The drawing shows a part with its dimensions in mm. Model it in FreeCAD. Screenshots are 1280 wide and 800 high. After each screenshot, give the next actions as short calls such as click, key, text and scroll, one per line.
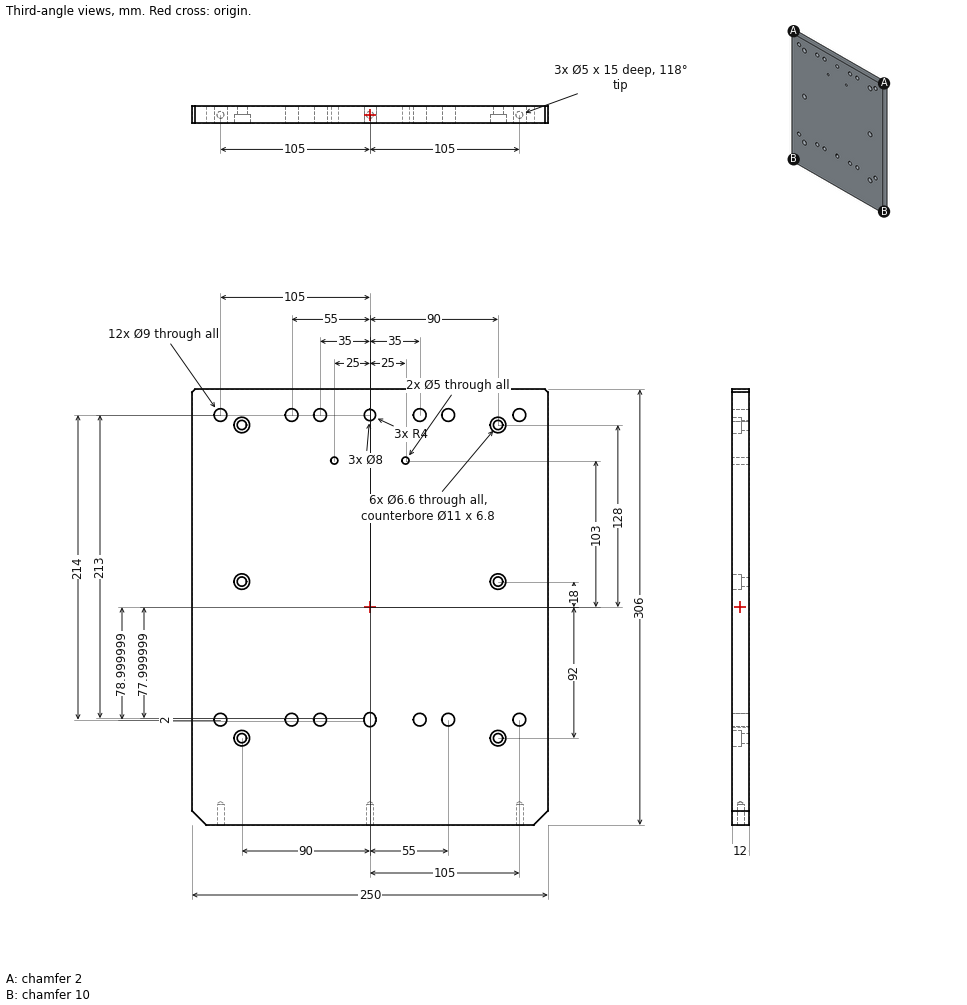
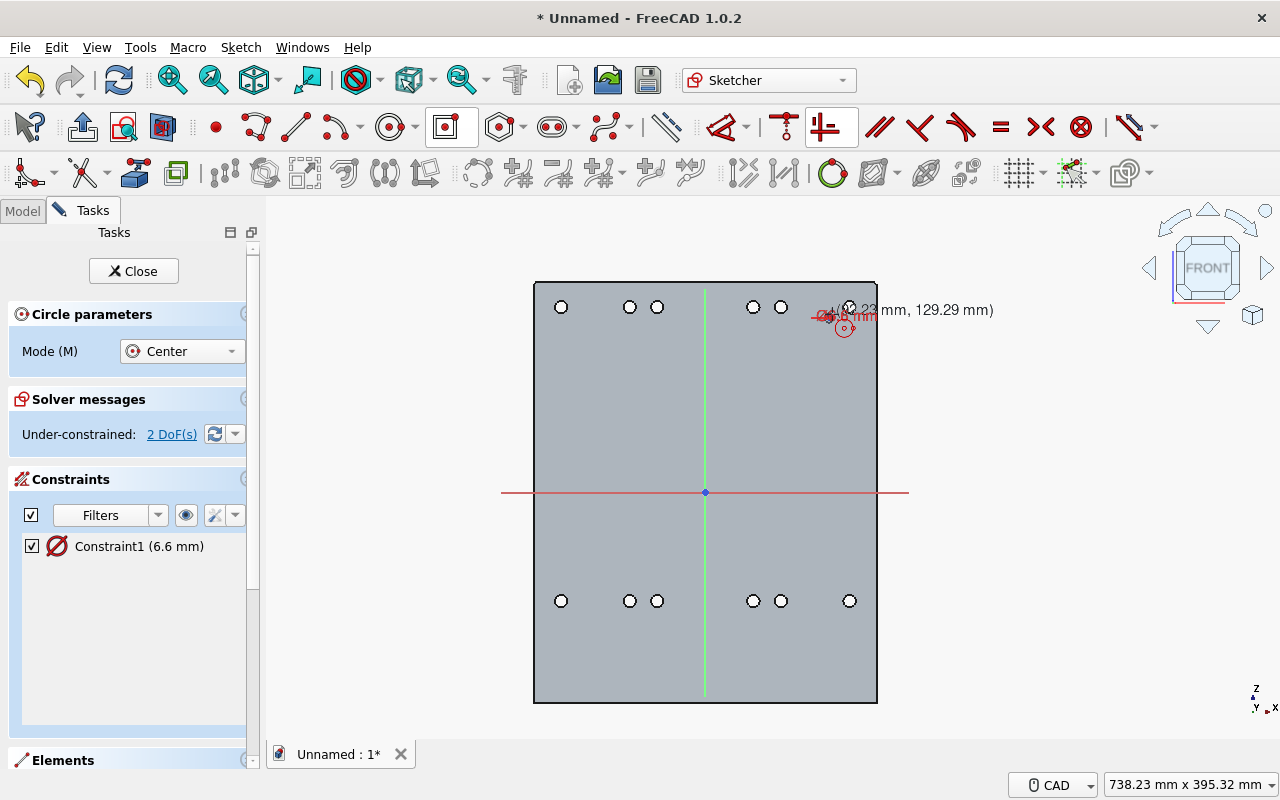
scroll(829, 468, up, 9)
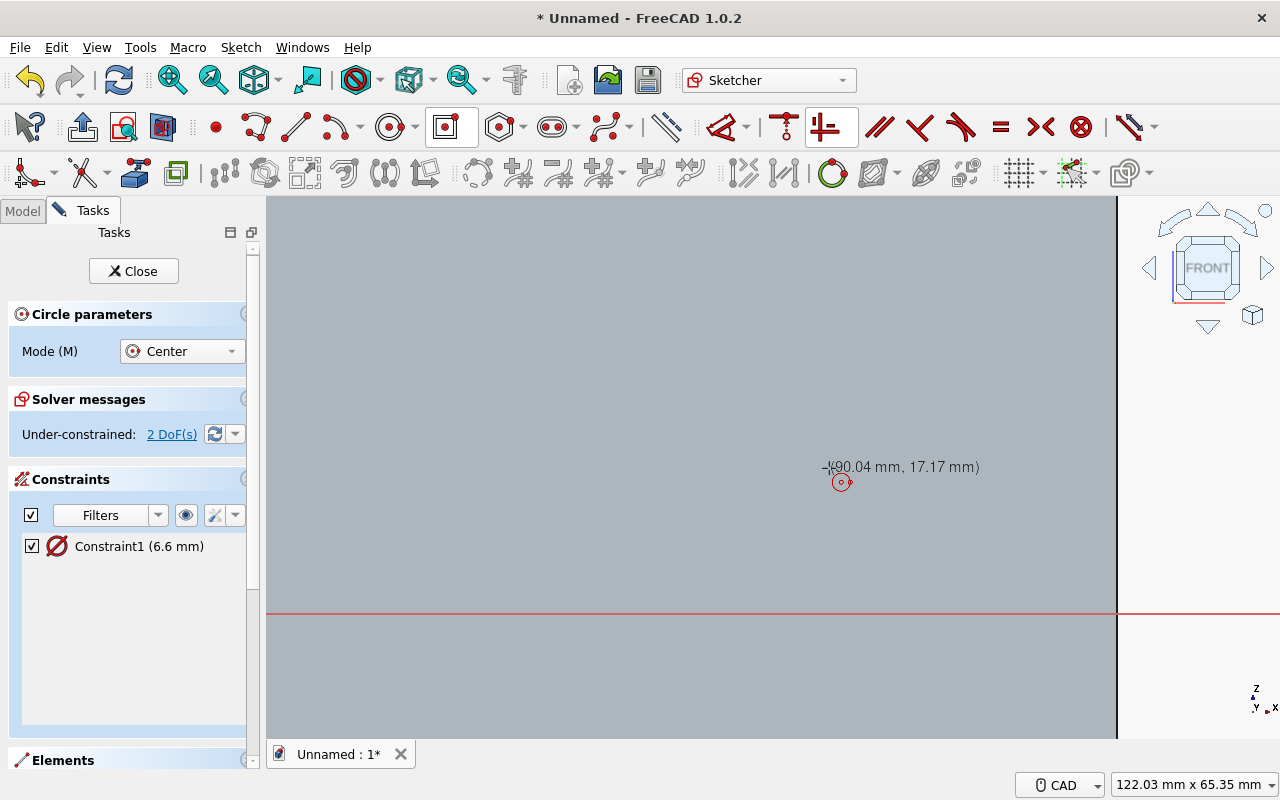
scroll(829, 468, down, 9)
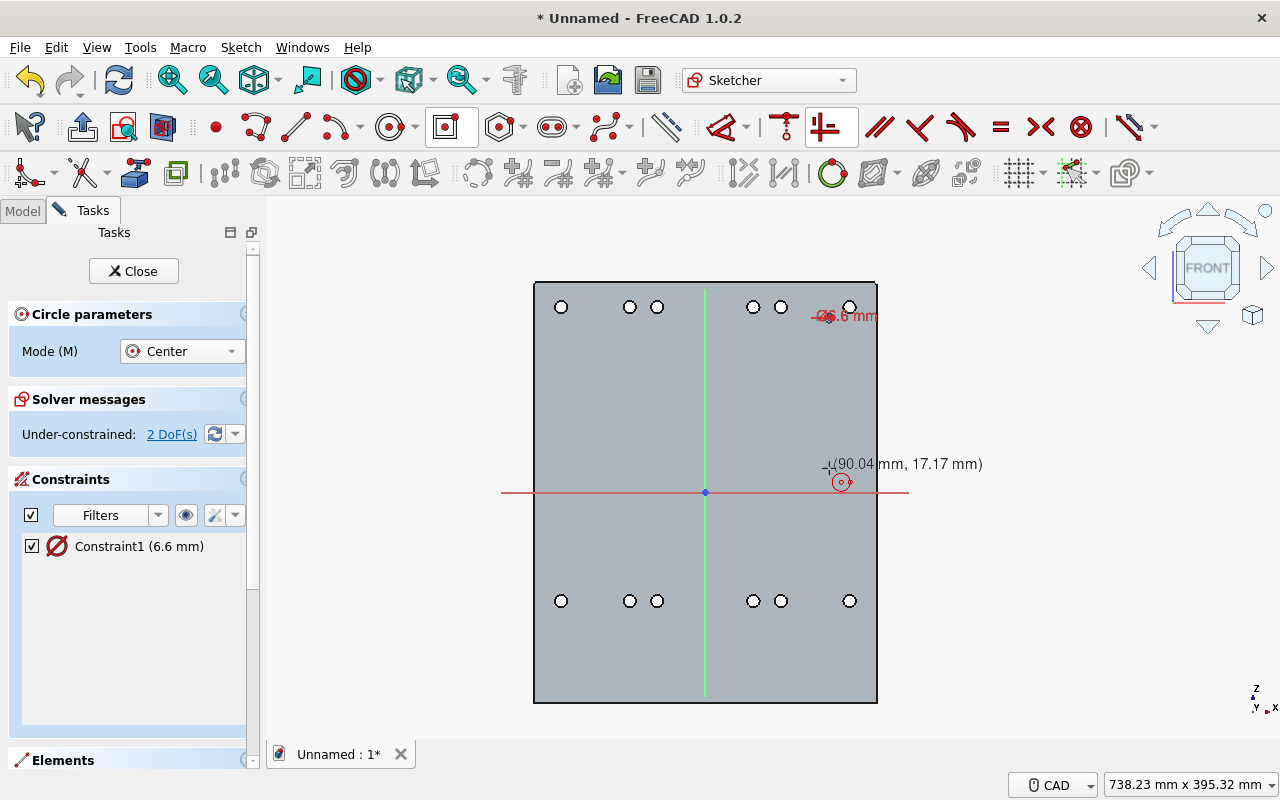
click(829, 468)
move(832, 465)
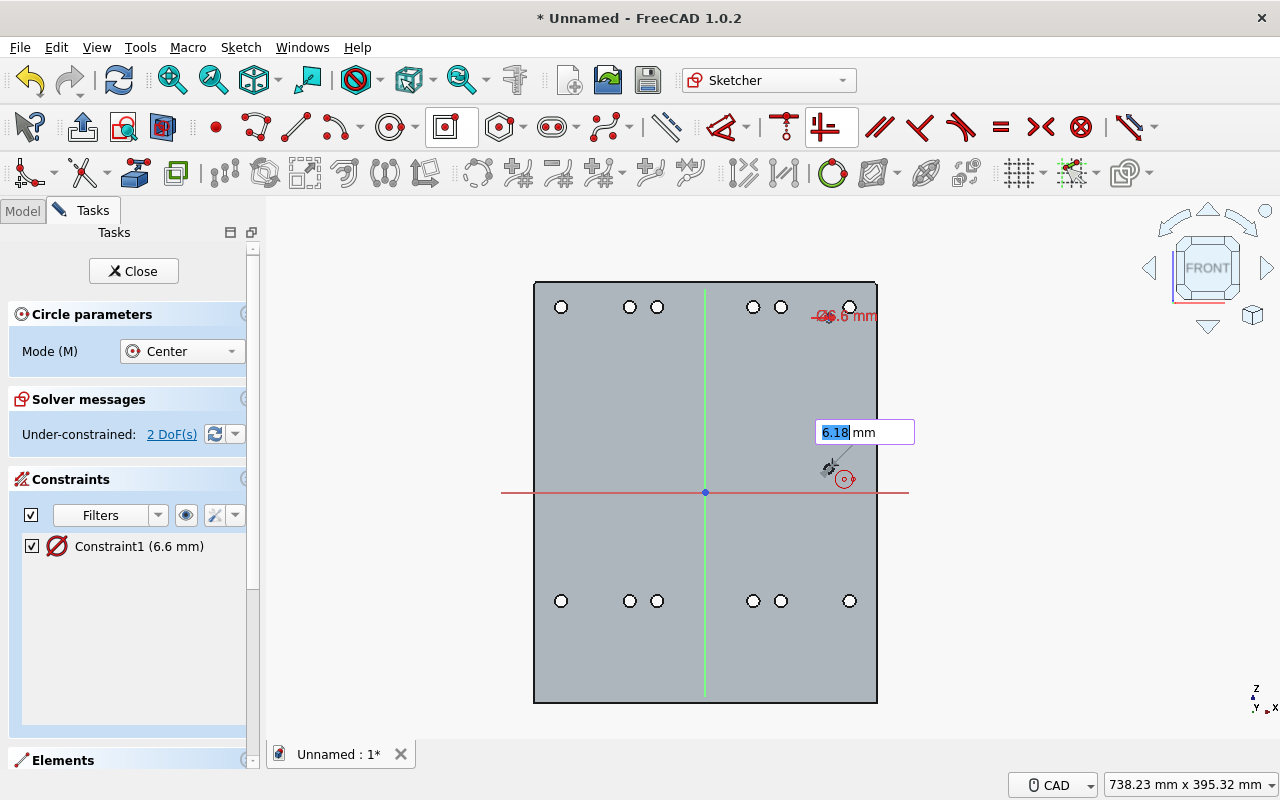
text(6.6)
key(Return)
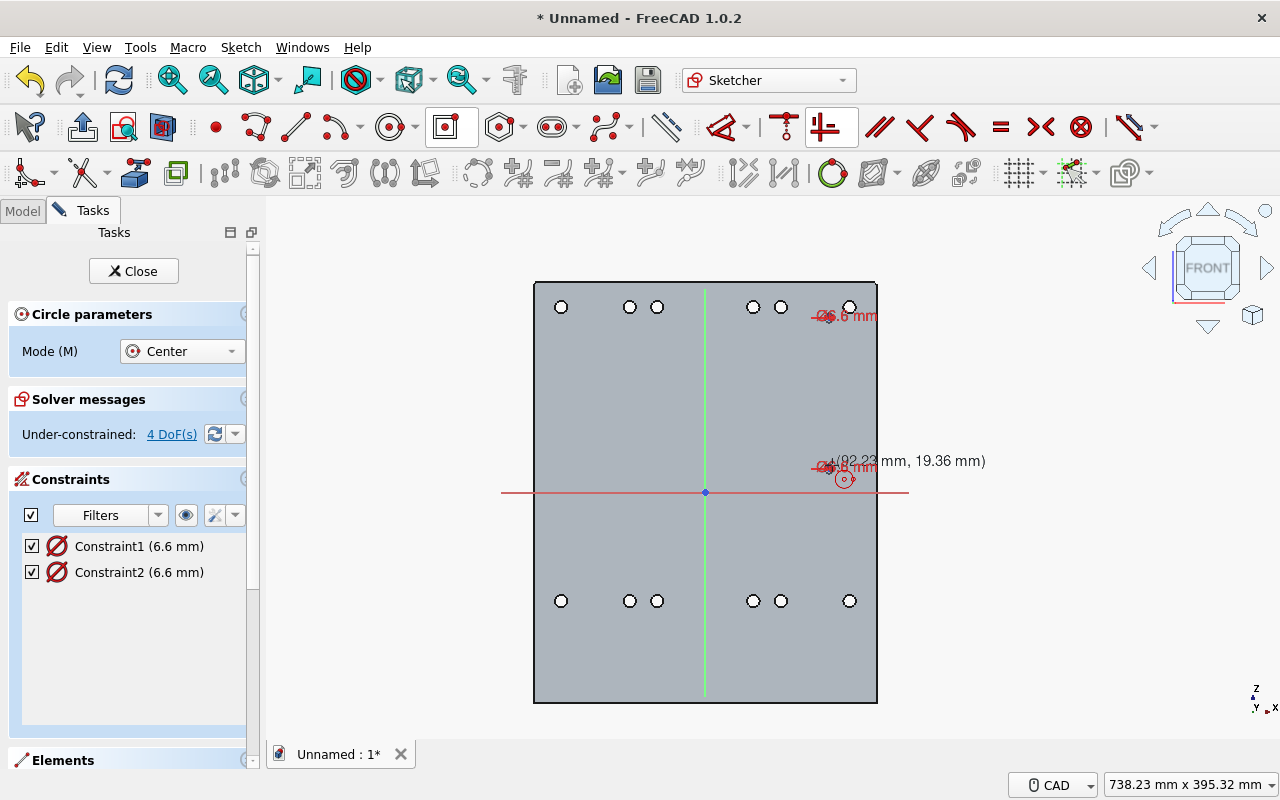
scroll(829, 619, up, 9)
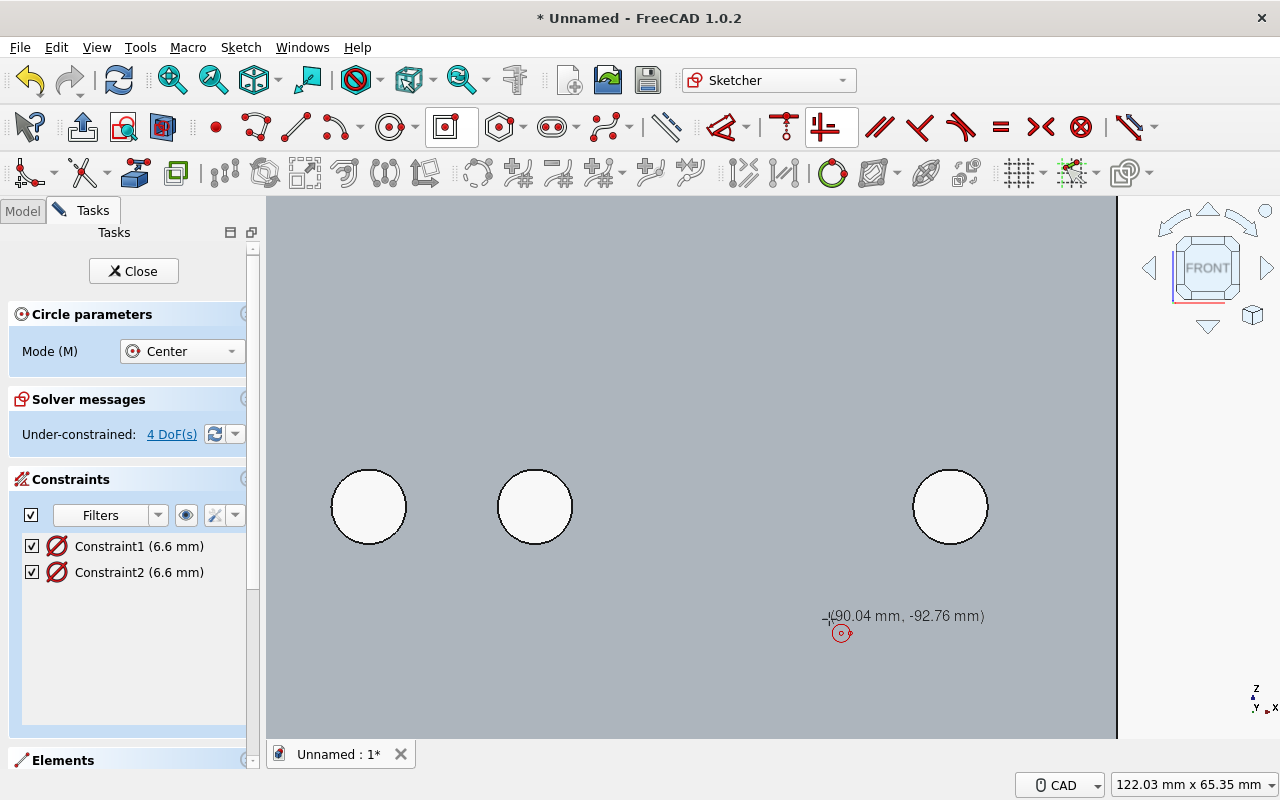
scroll(829, 619, down, 9)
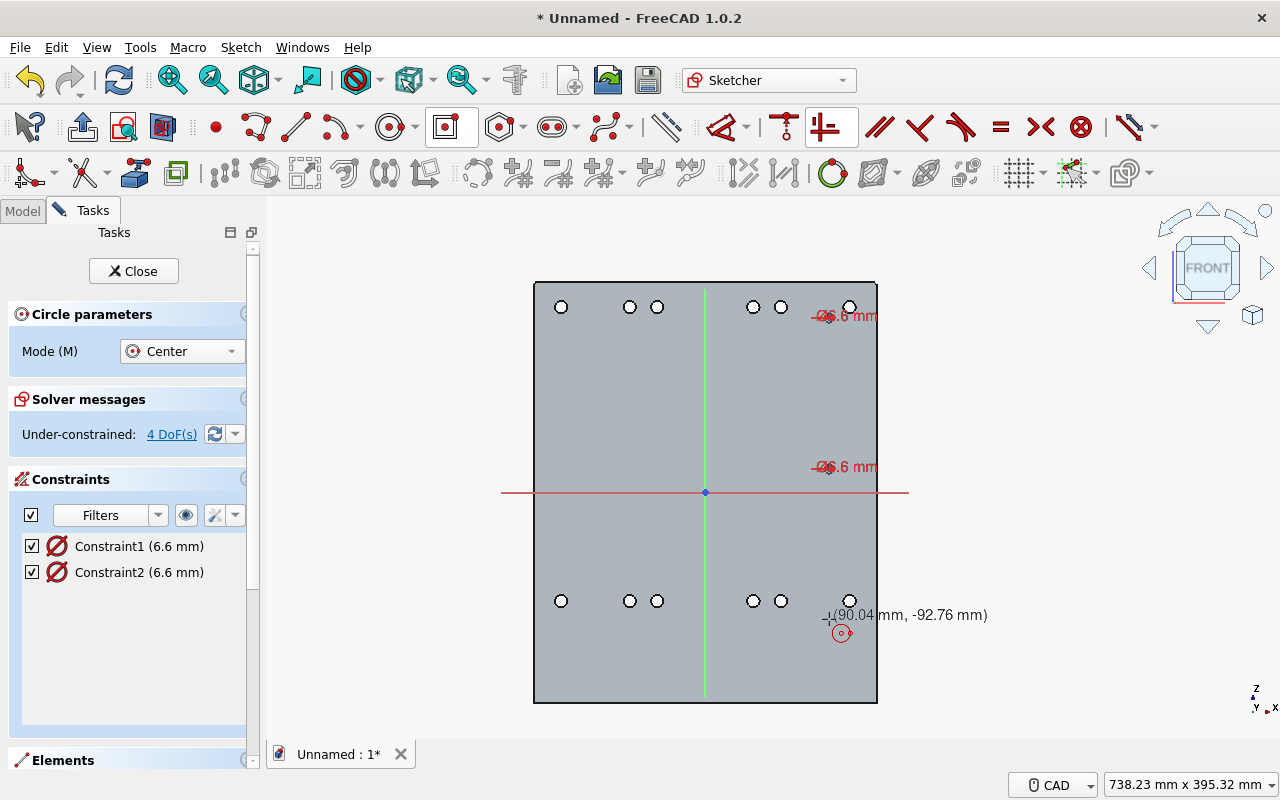
click(829, 619)
move(832, 616)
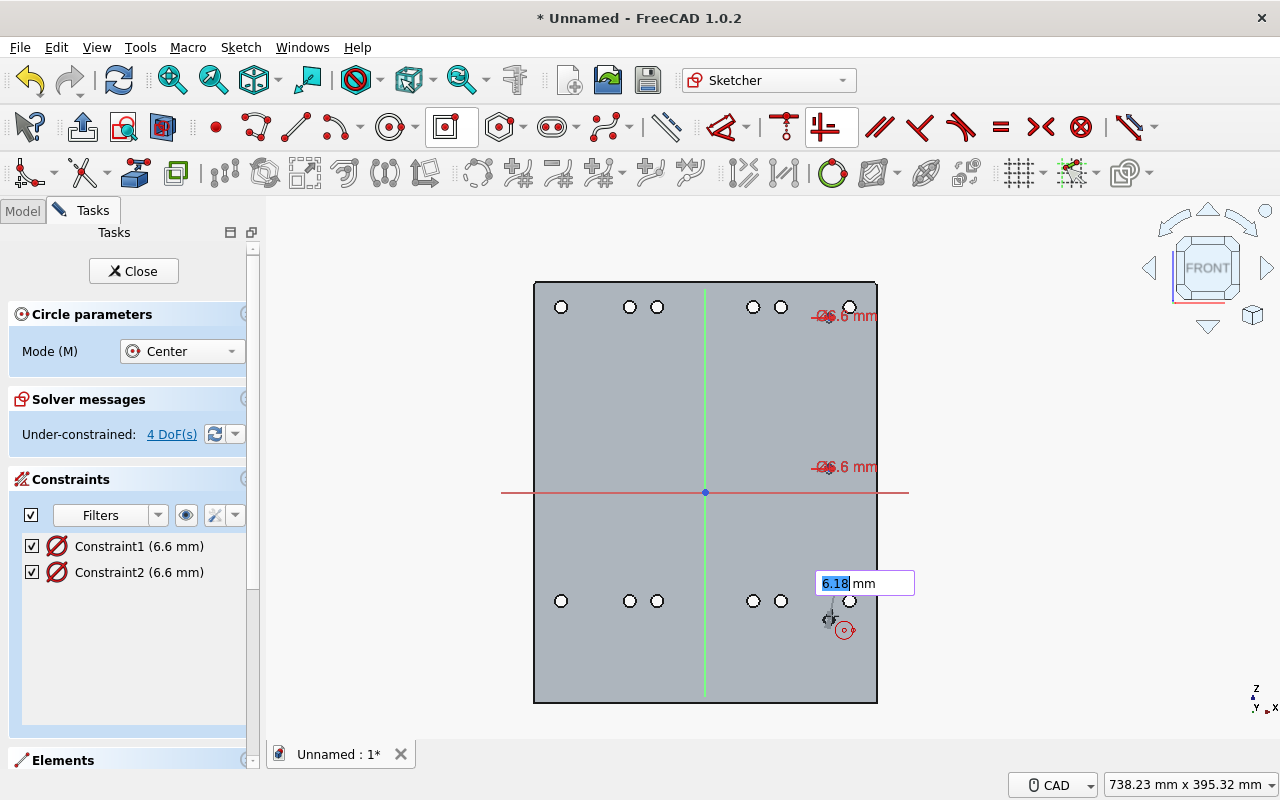
text(6.6)
key(Return)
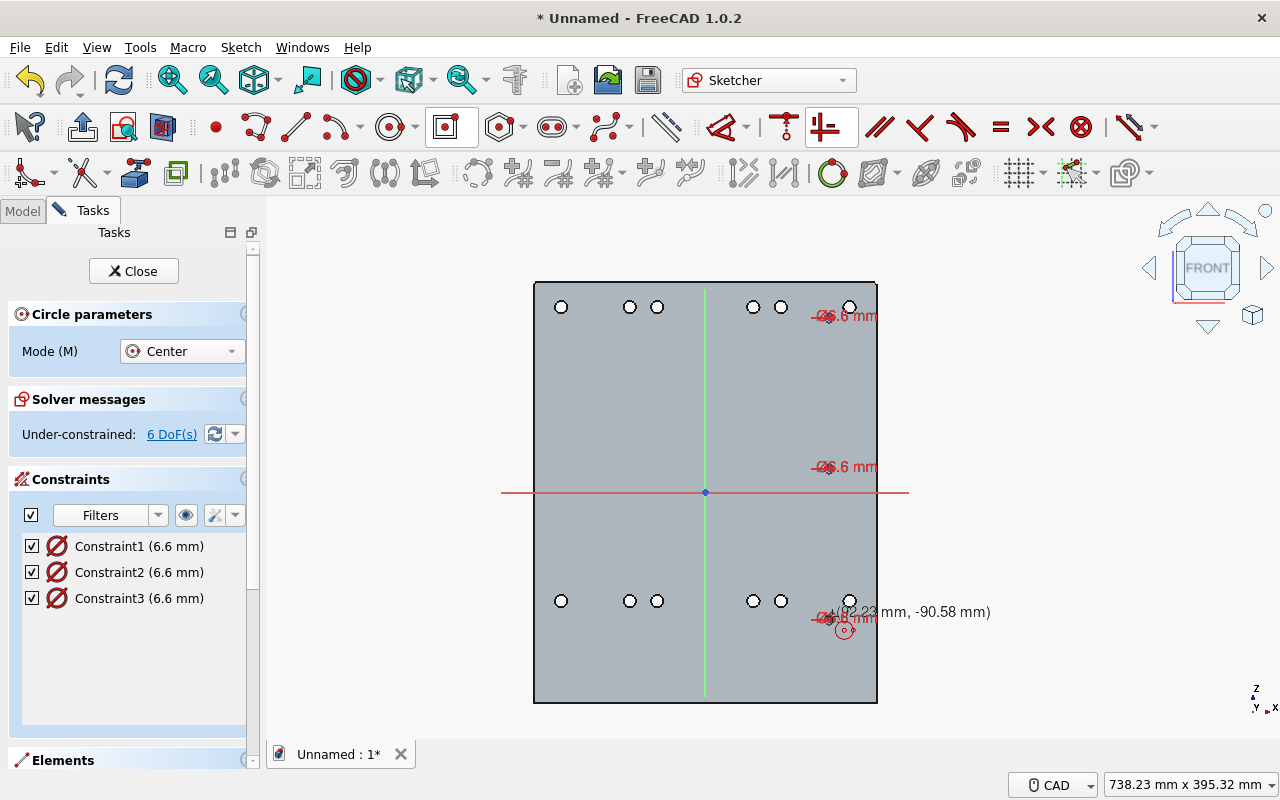
scroll(582, 619, up, 9)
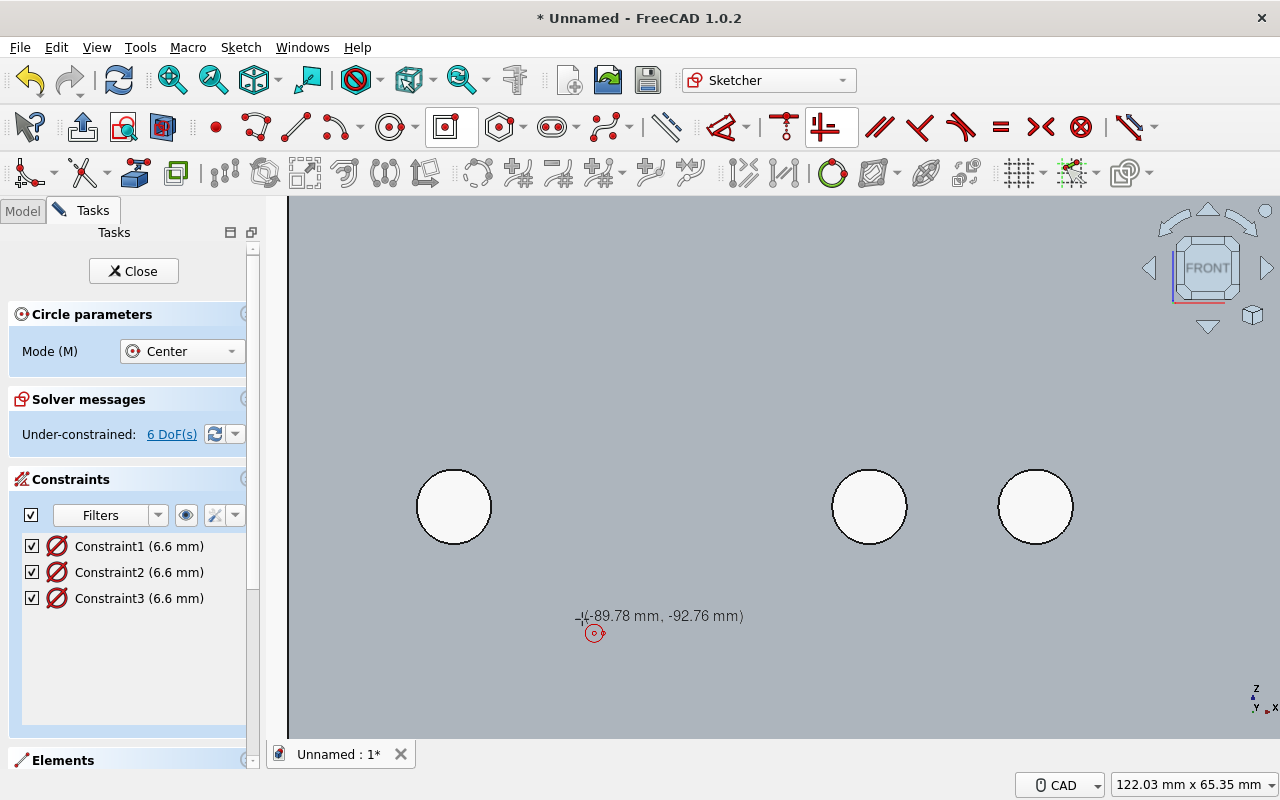
scroll(581, 619, down, 9)